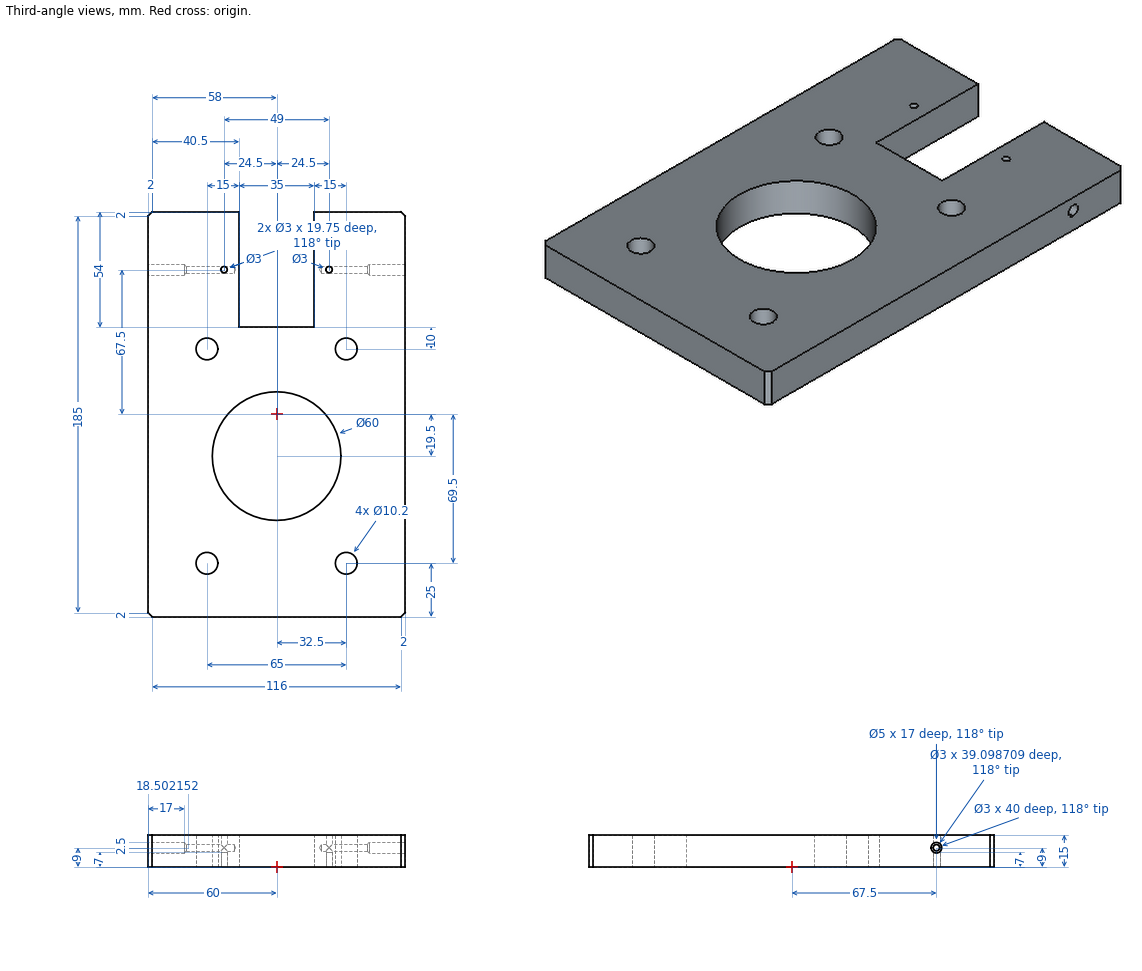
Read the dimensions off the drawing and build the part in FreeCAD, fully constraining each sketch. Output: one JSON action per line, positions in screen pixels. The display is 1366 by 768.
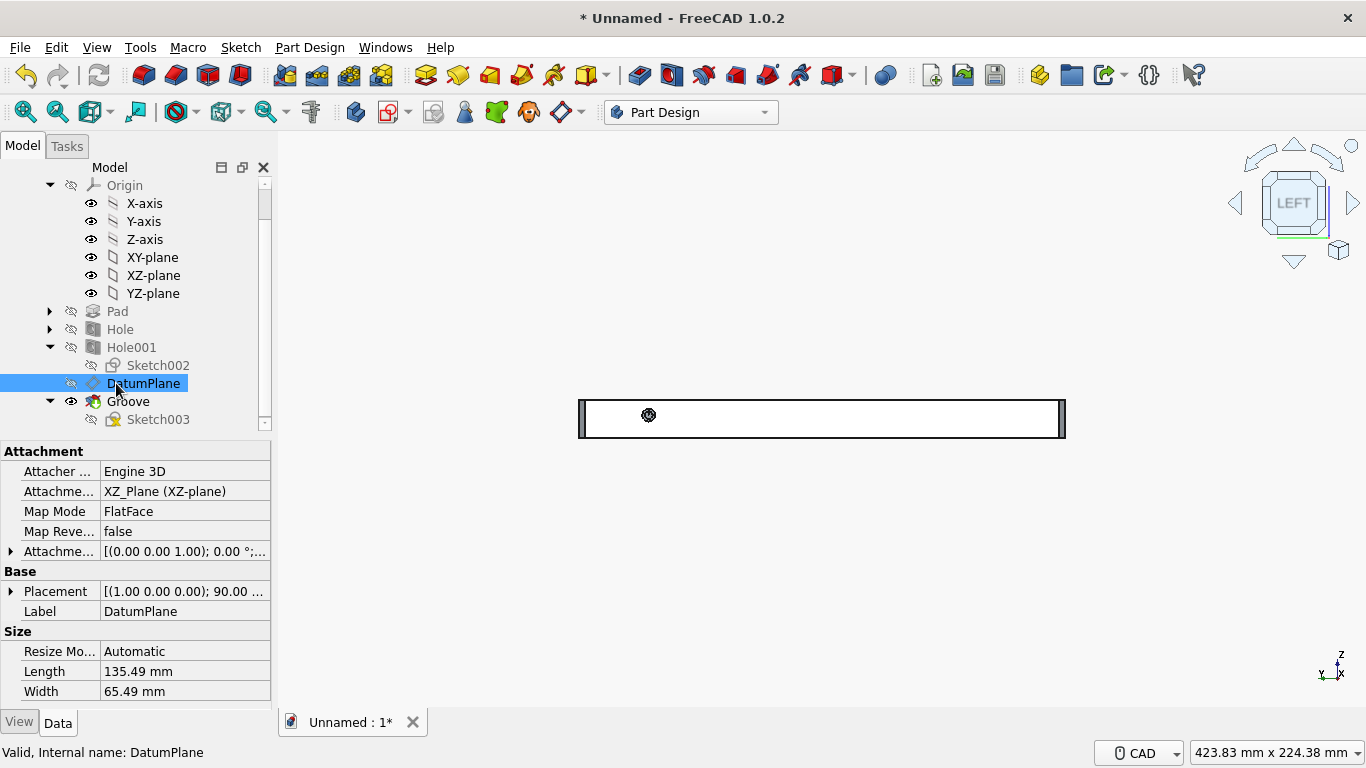
{"action": "key", "text": "0"}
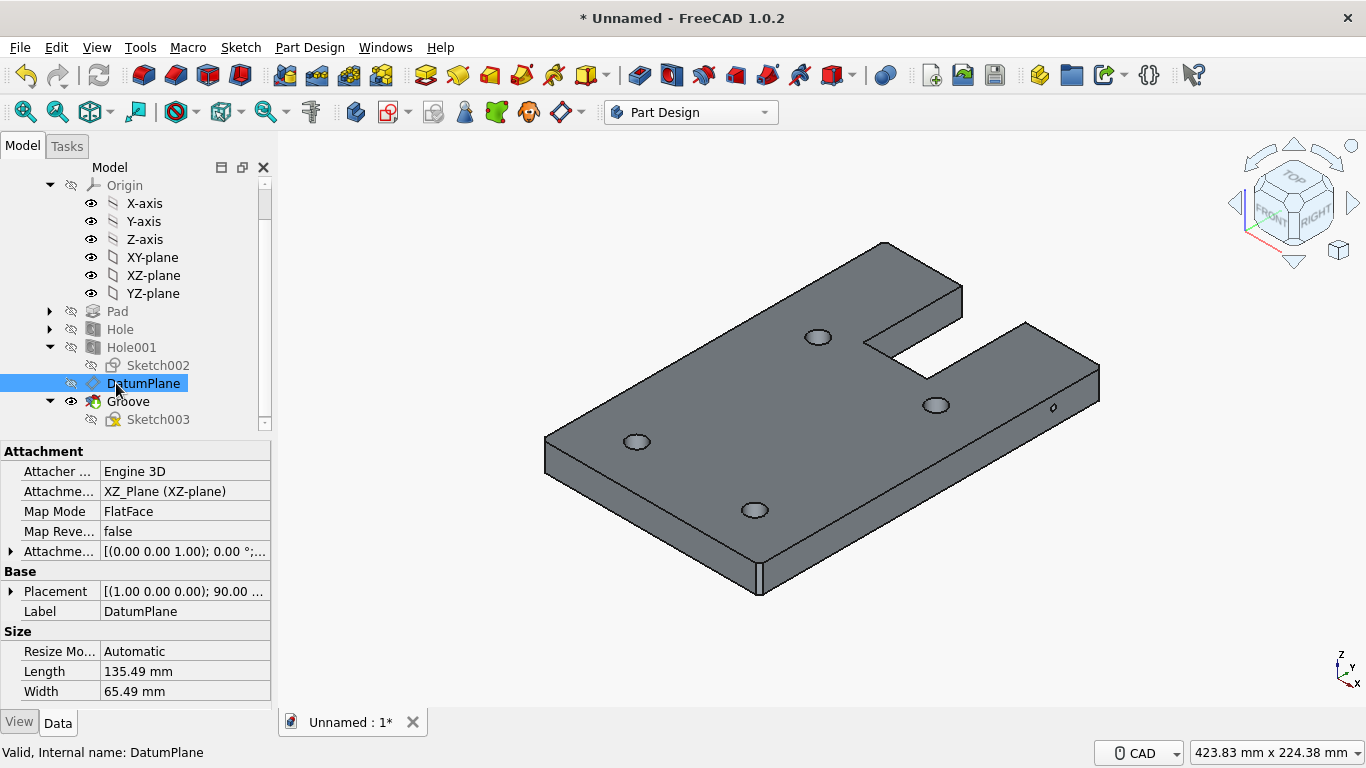
{"action": "left_click", "coordinate": [1075, 398]}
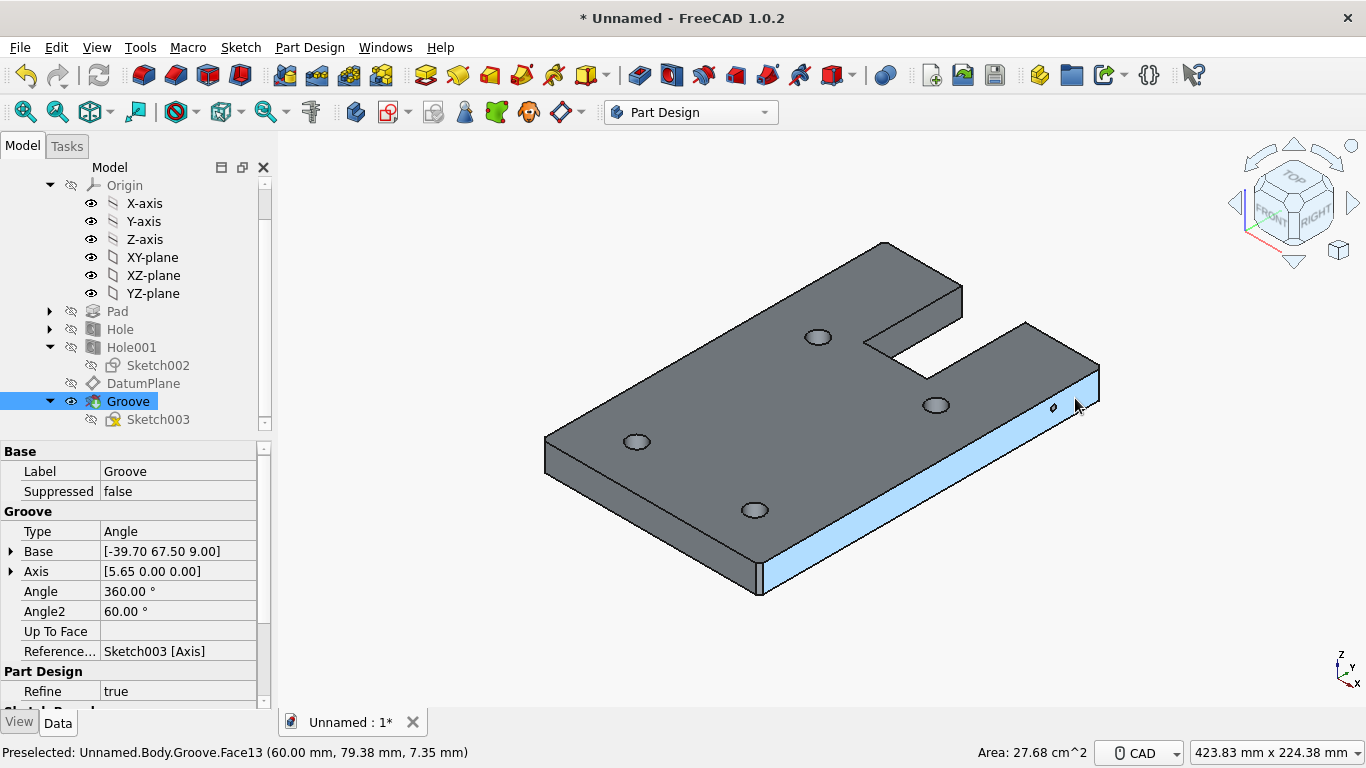
{"action": "left_click", "coordinate": [388, 112]}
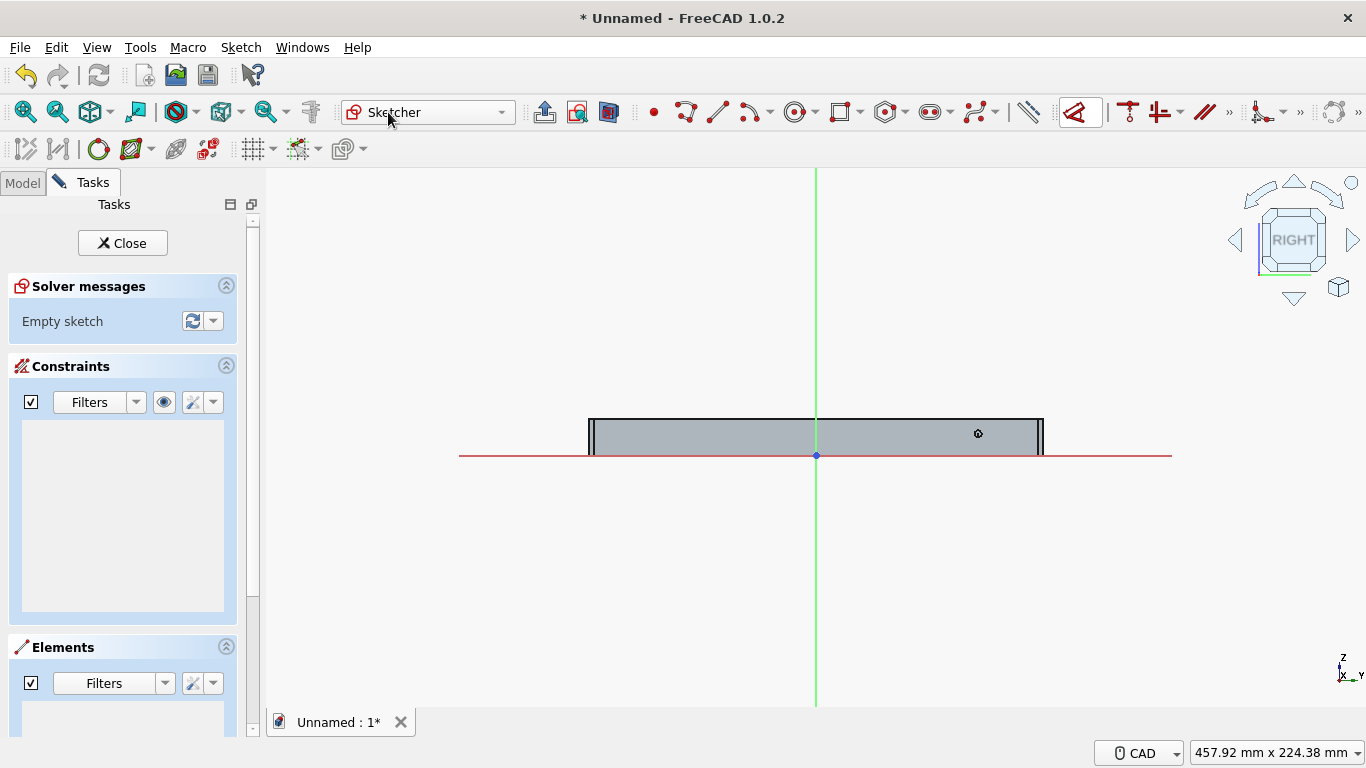
{"action": "scroll", "coordinate": [990, 434], "scroll_direction": "up", "scroll_amount": 15}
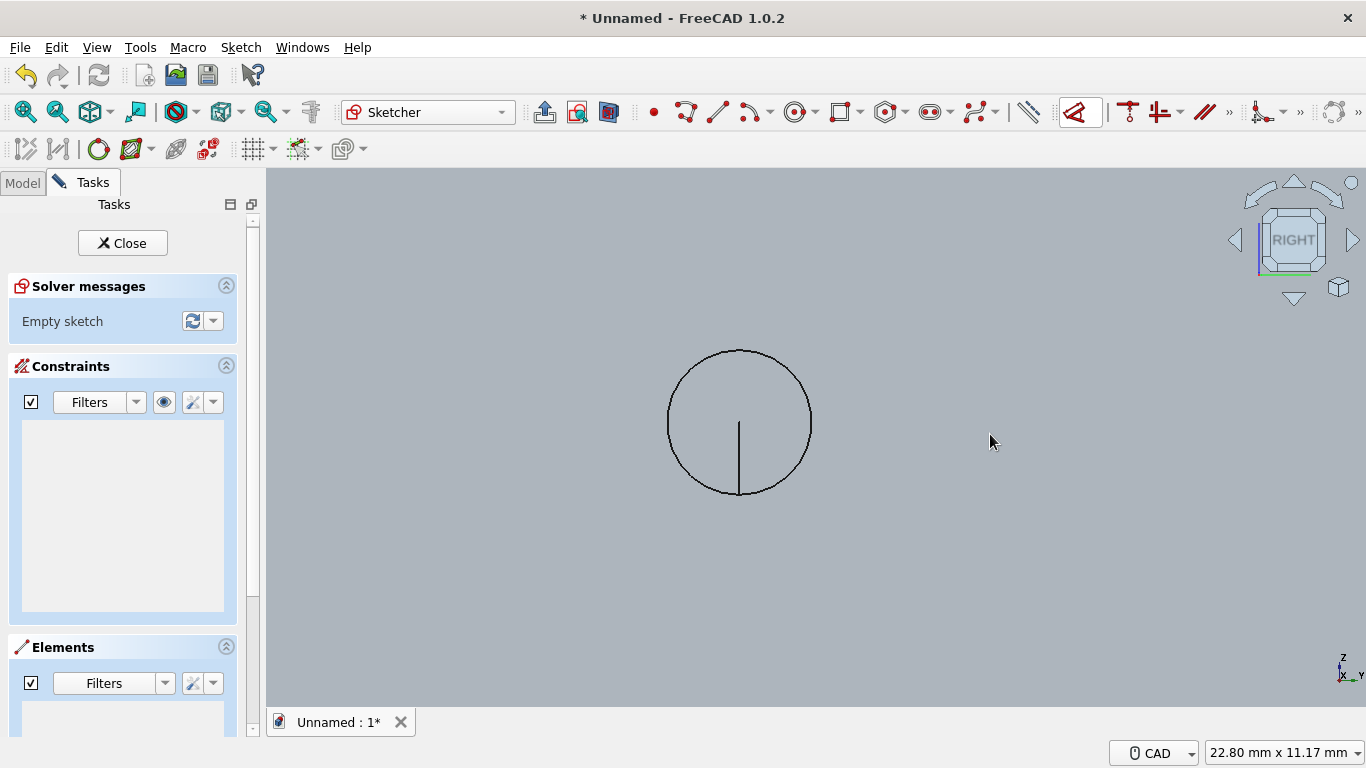
{"action": "scroll", "coordinate": [723, 392], "scroll_direction": "up", "scroll_amount": 2}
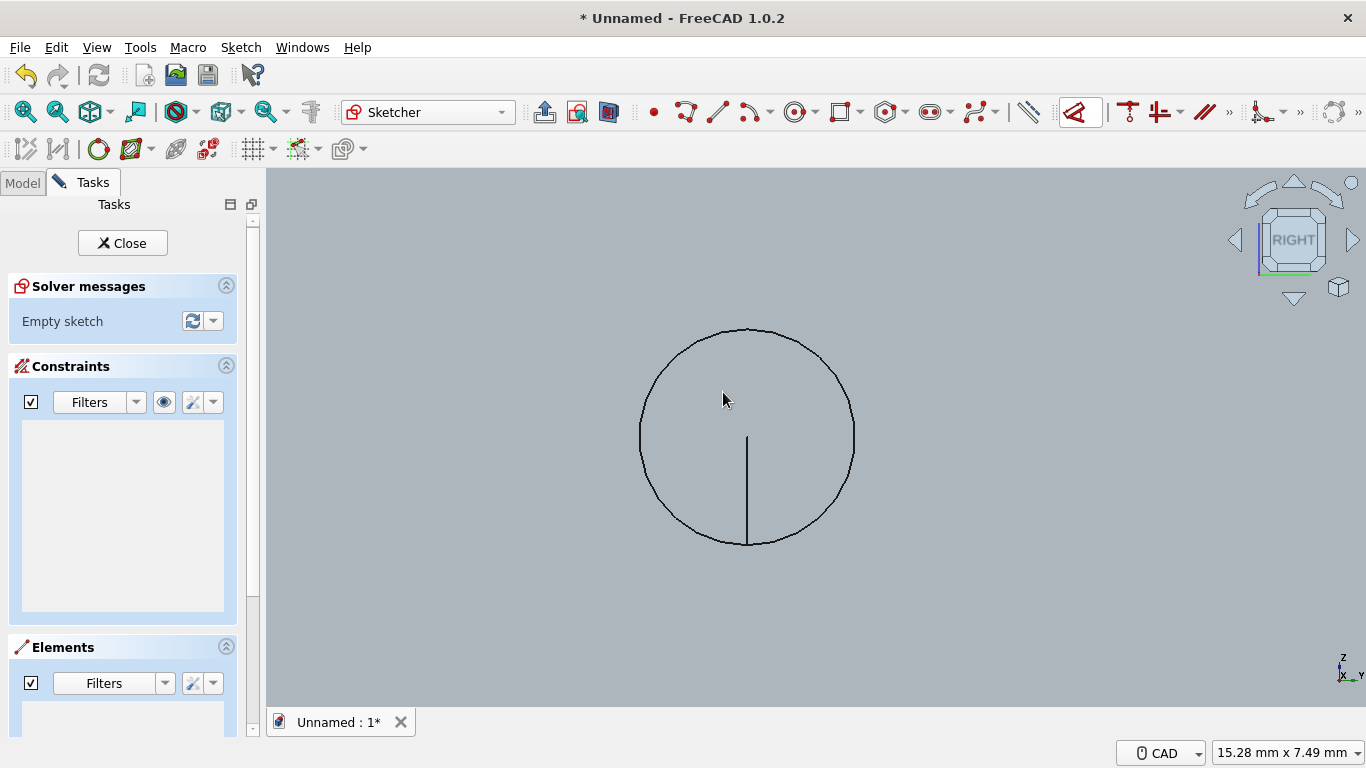
{"action": "left_click", "coordinate": [796, 112]}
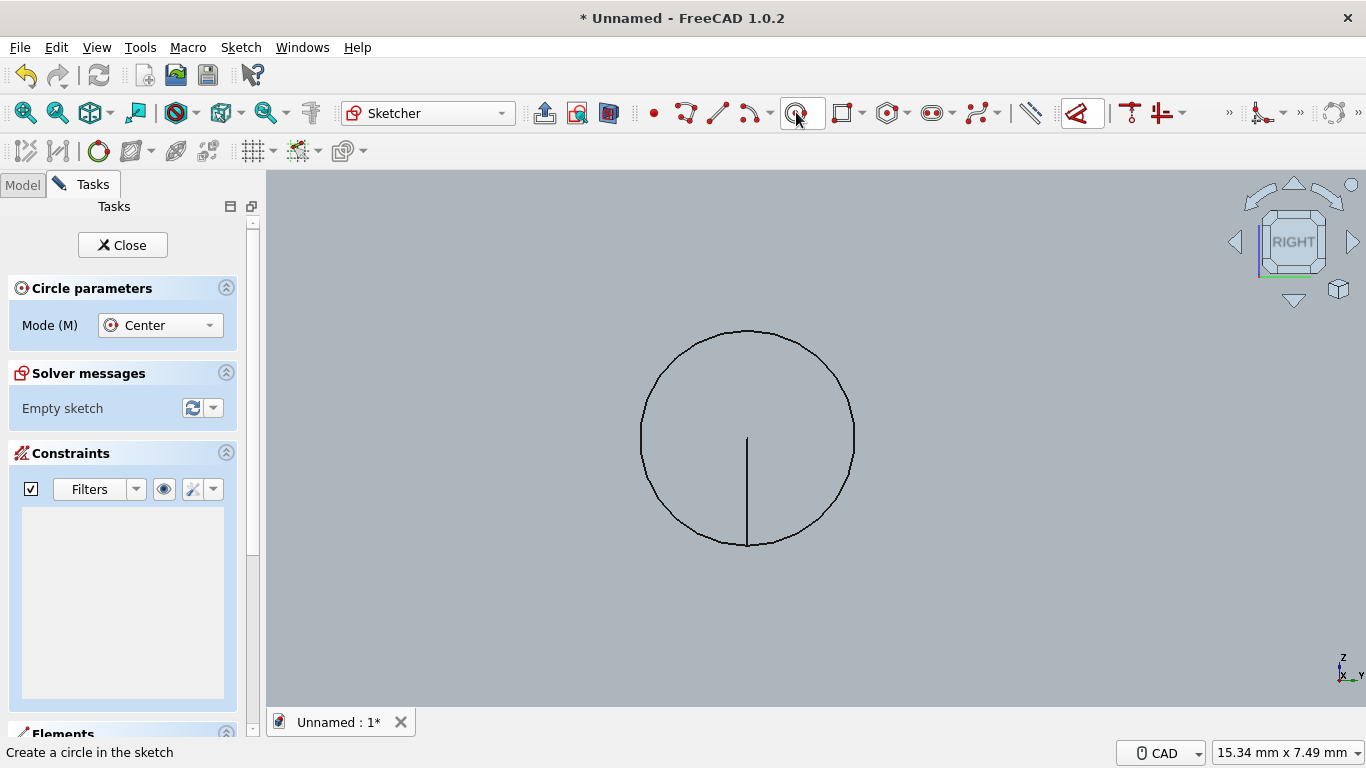
{"action": "left_click", "coordinate": [747, 438]}
{"action": "mouse_move", "coordinate": [874, 312]}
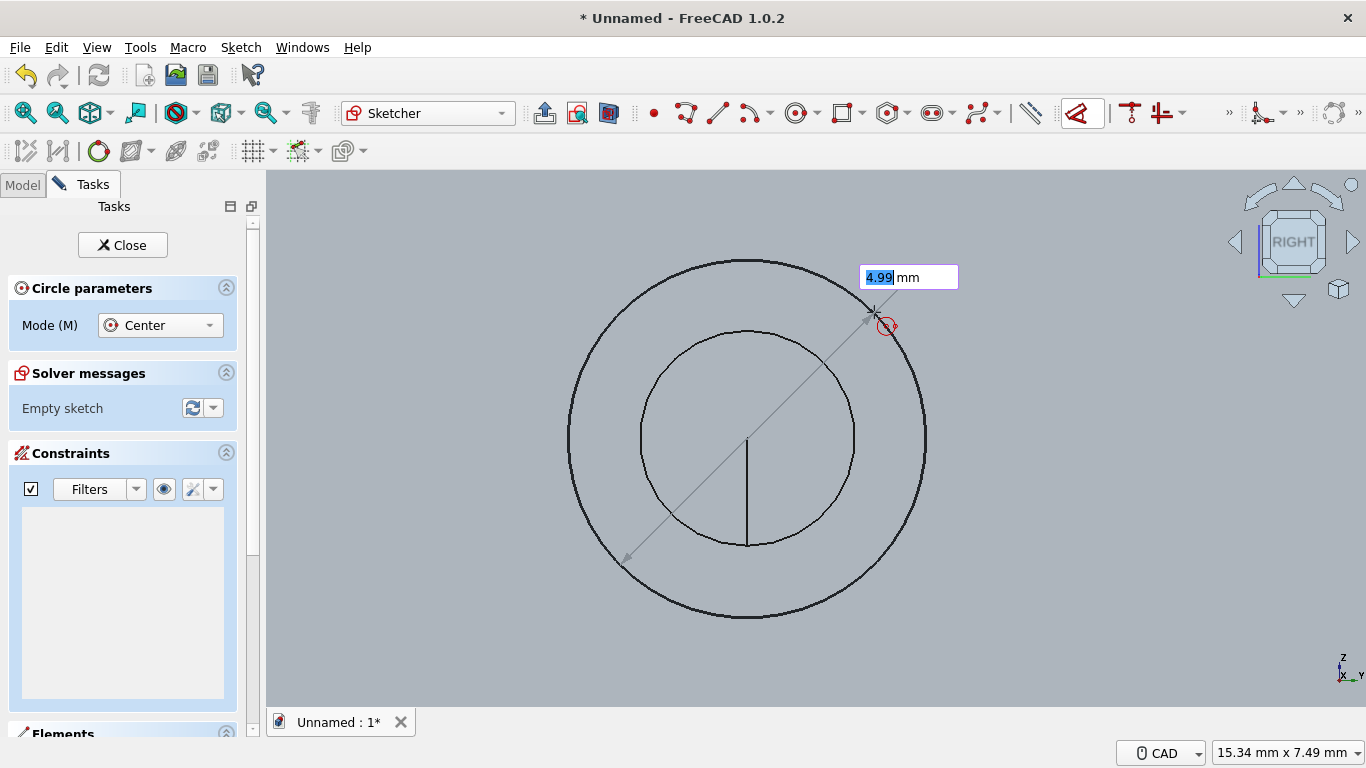
{"action": "type", "text": "5"}
{"action": "key", "text": "Return"}
{"action": "key", "text": "Escape"}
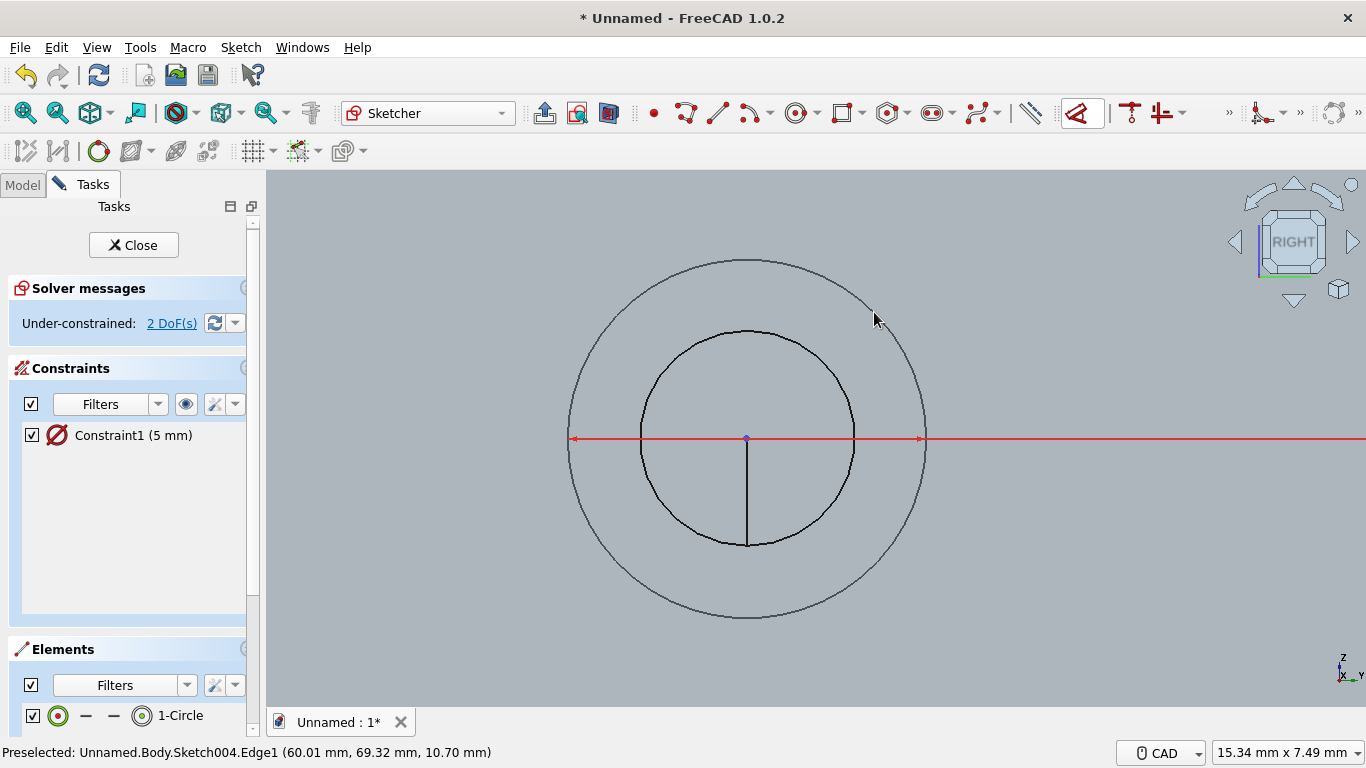
{"action": "left_click", "coordinate": [747, 439]}